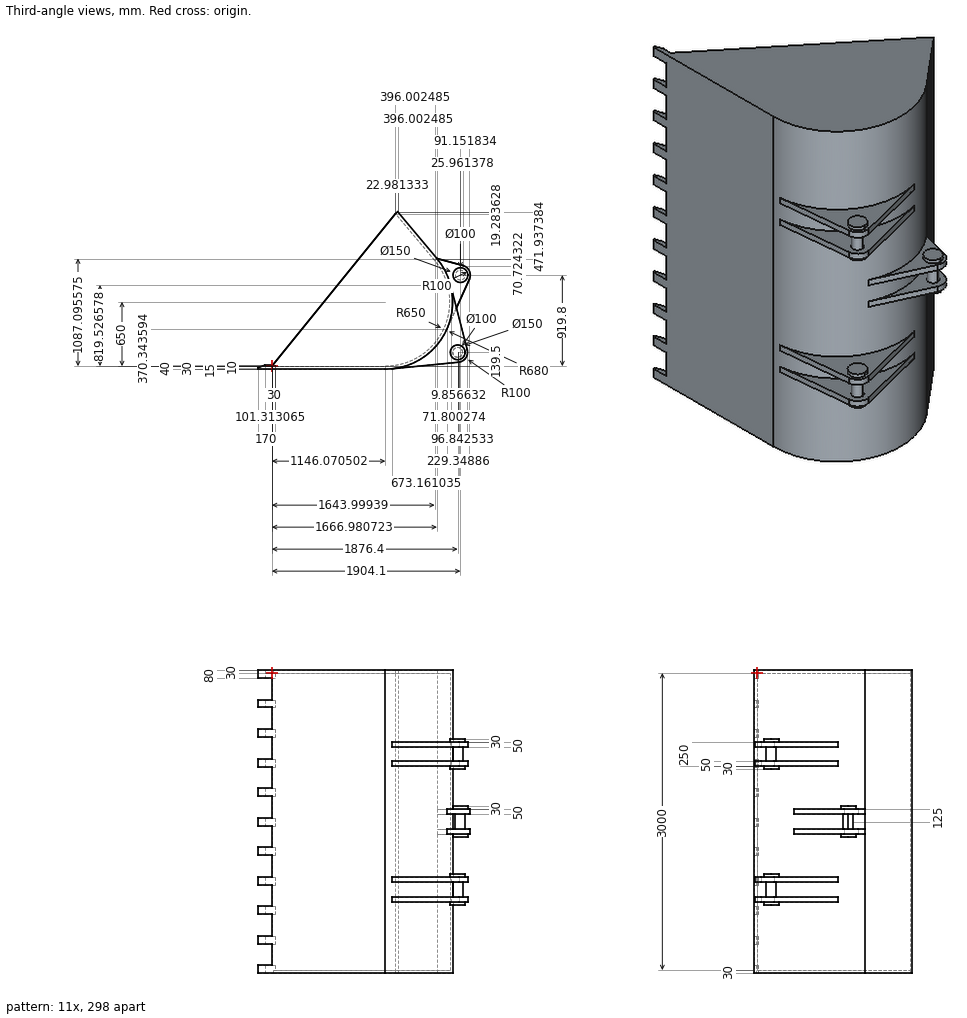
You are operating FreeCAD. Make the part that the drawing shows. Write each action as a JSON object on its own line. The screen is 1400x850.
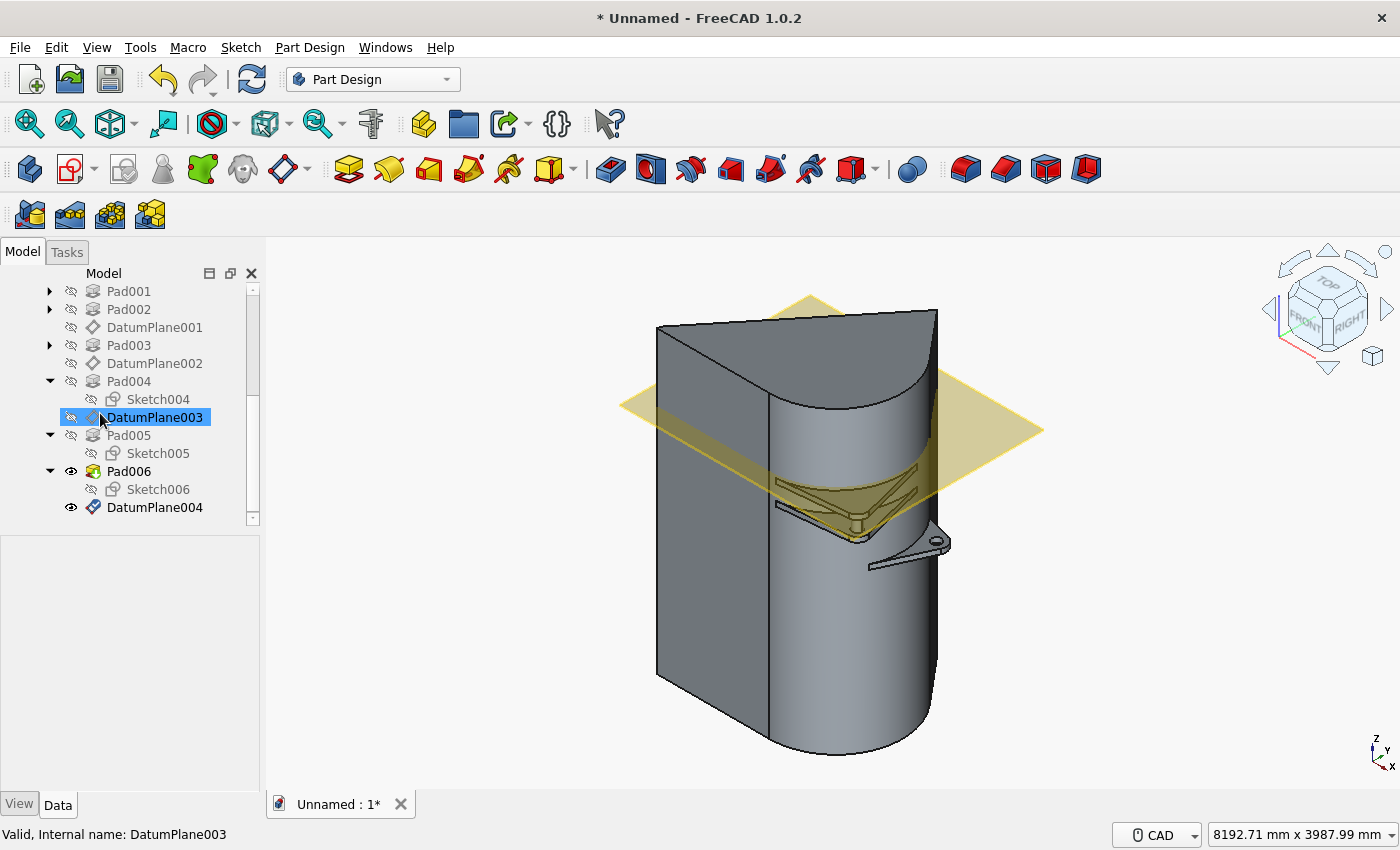
{"action": "left_click", "coordinate": [116, 507]}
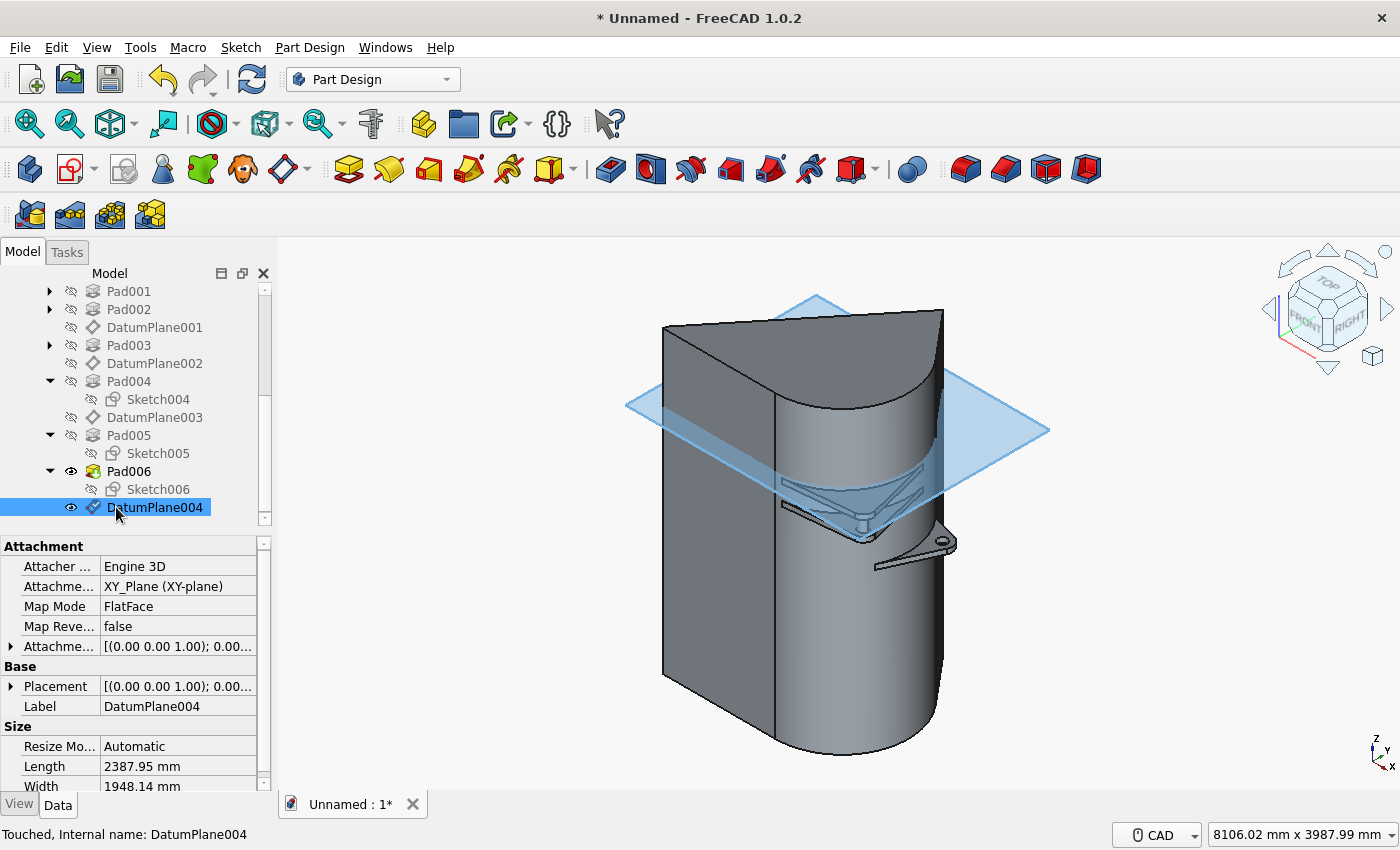
{"action": "left_click", "coordinate": [70, 170]}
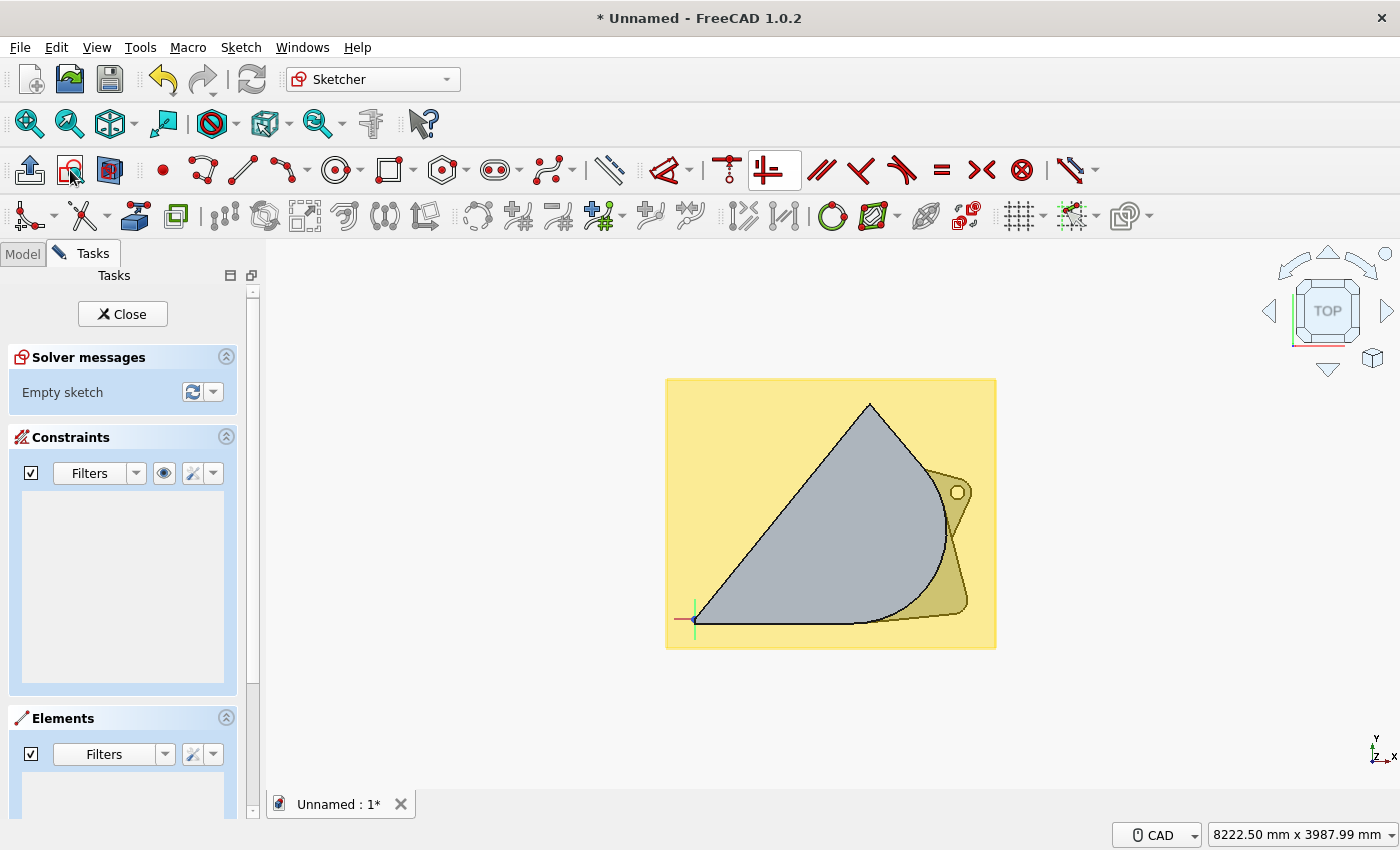
{"action": "key", "text": "q s"}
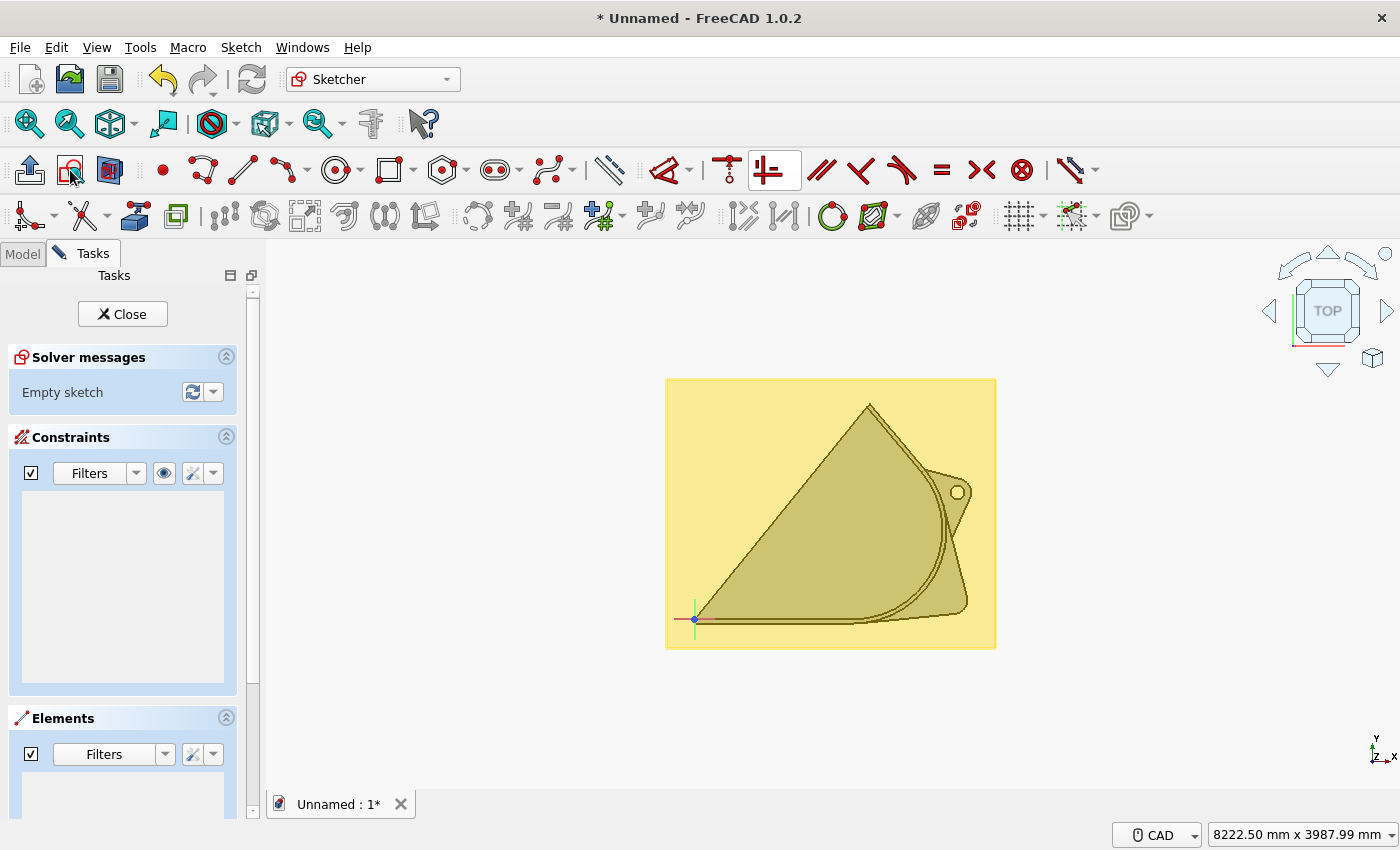
{"action": "scroll", "coordinate": [966, 606], "scroll_direction": "up", "scroll_amount": 14}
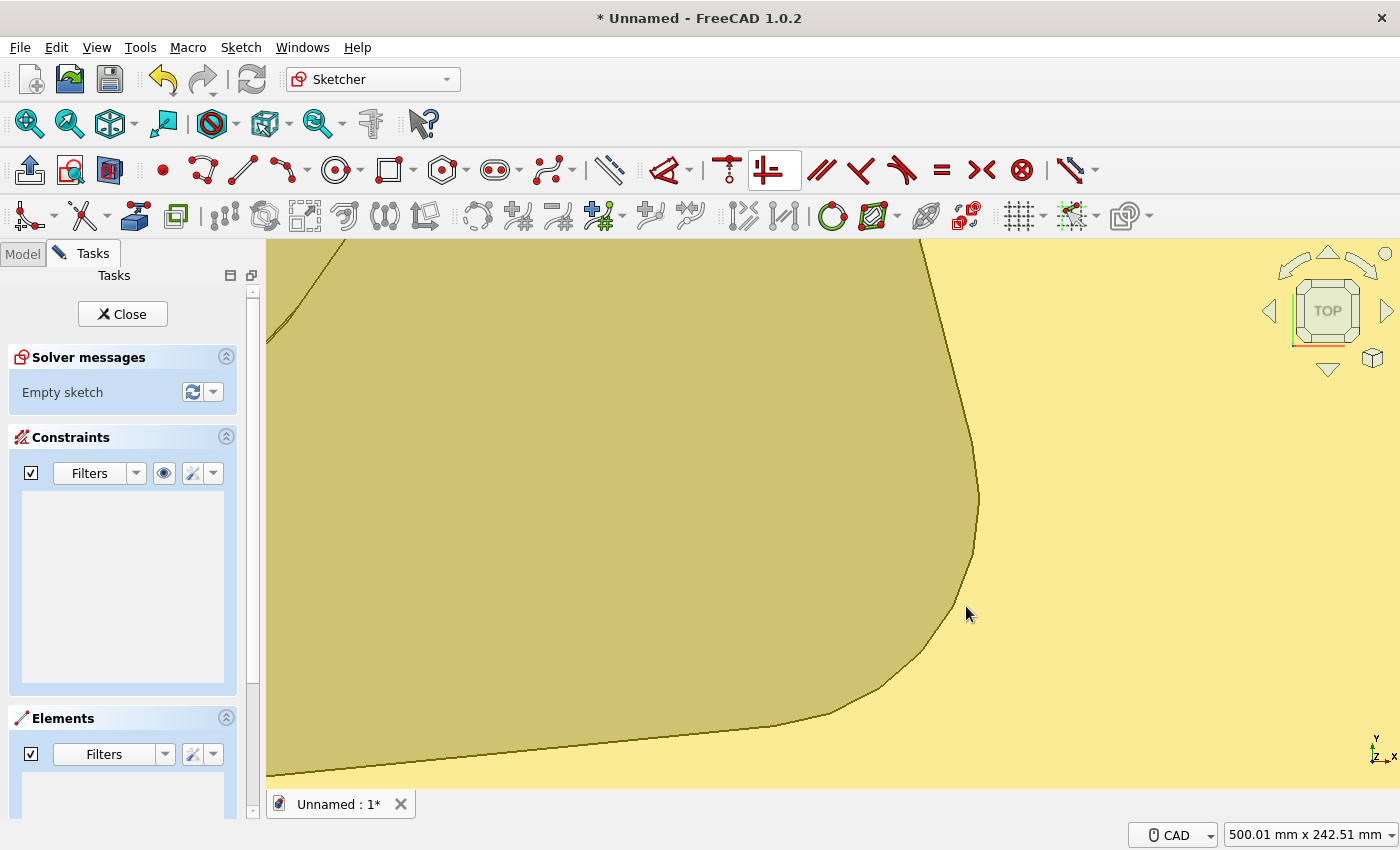
{"action": "left_click", "coordinate": [336, 170]}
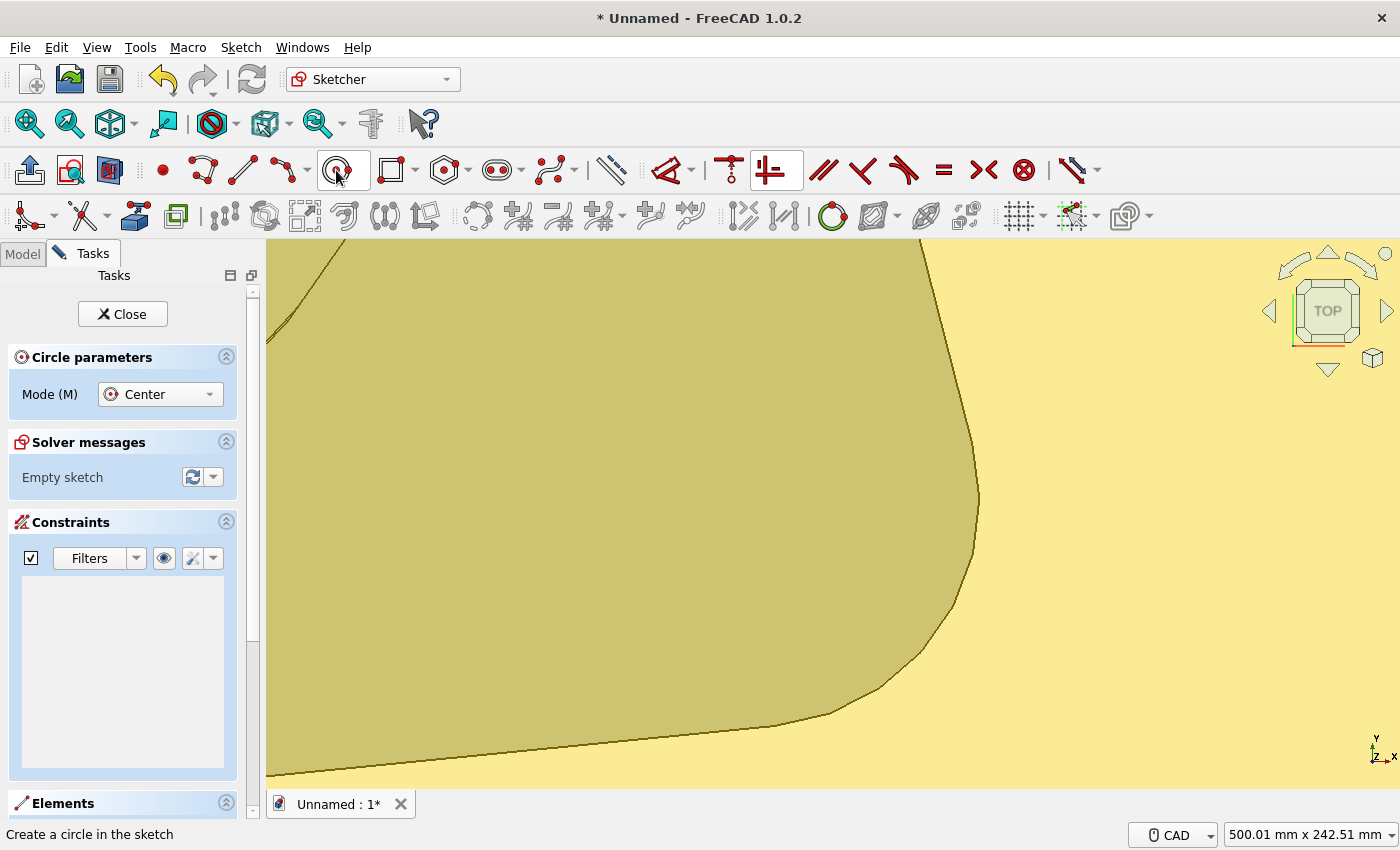
{"action": "left_click", "coordinate": [753, 500]}
{"action": "left_click", "coordinate": [873, 380]}
{"action": "key", "text": "Escape"}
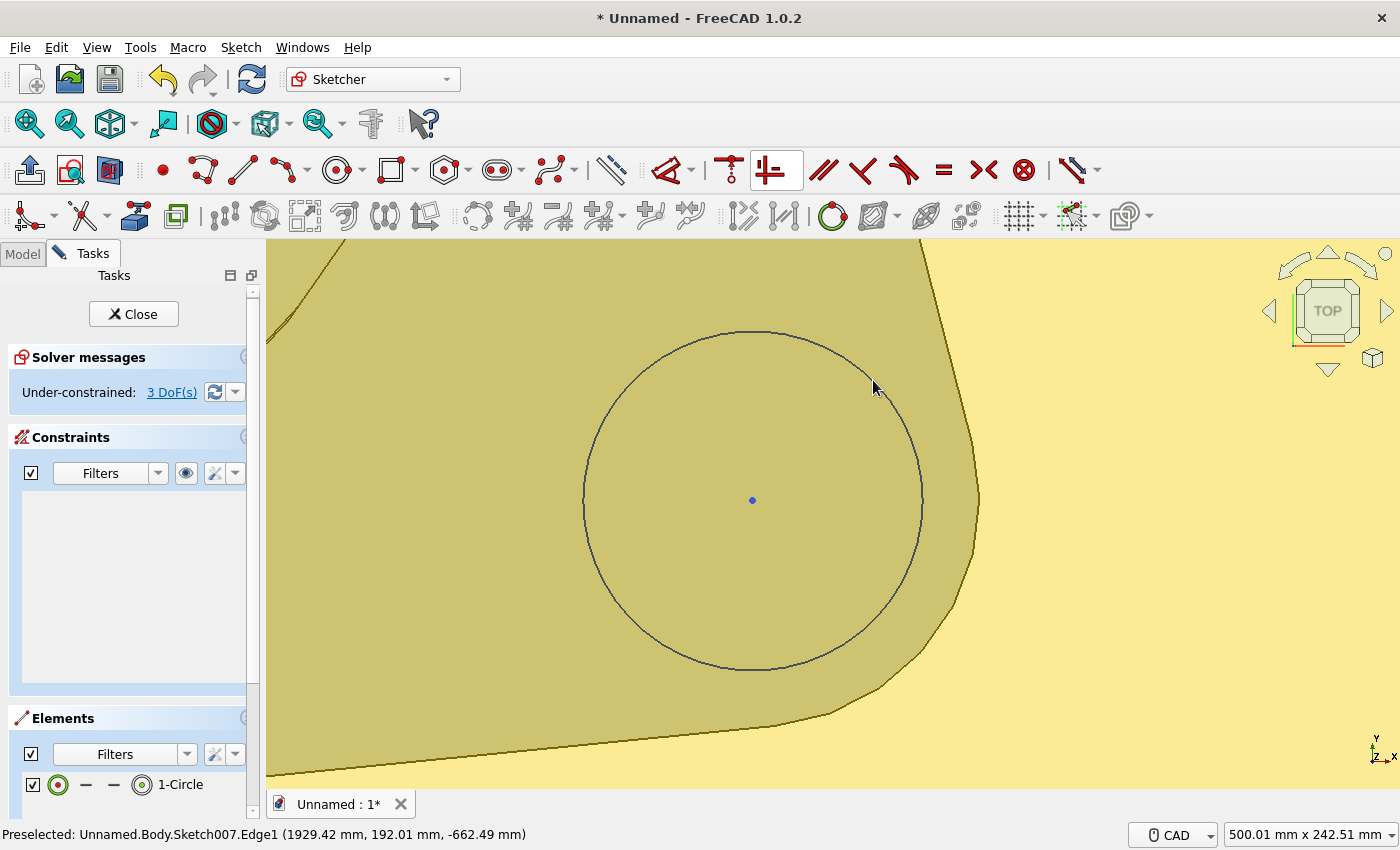
{"action": "left_click", "coordinate": [666, 170]}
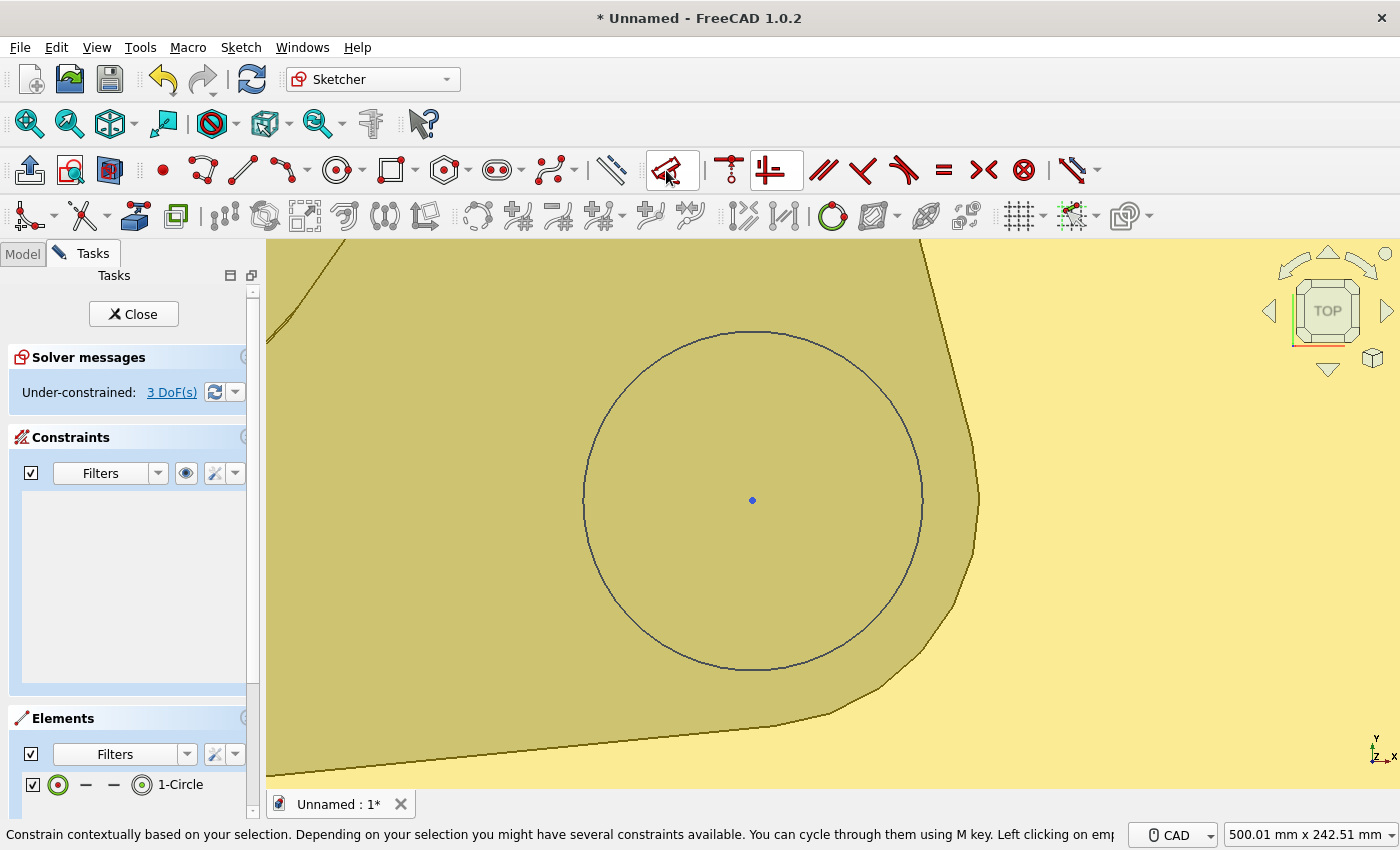
{"action": "left_click", "coordinate": [873, 381]}
{"action": "left_click", "coordinate": [896, 358]}